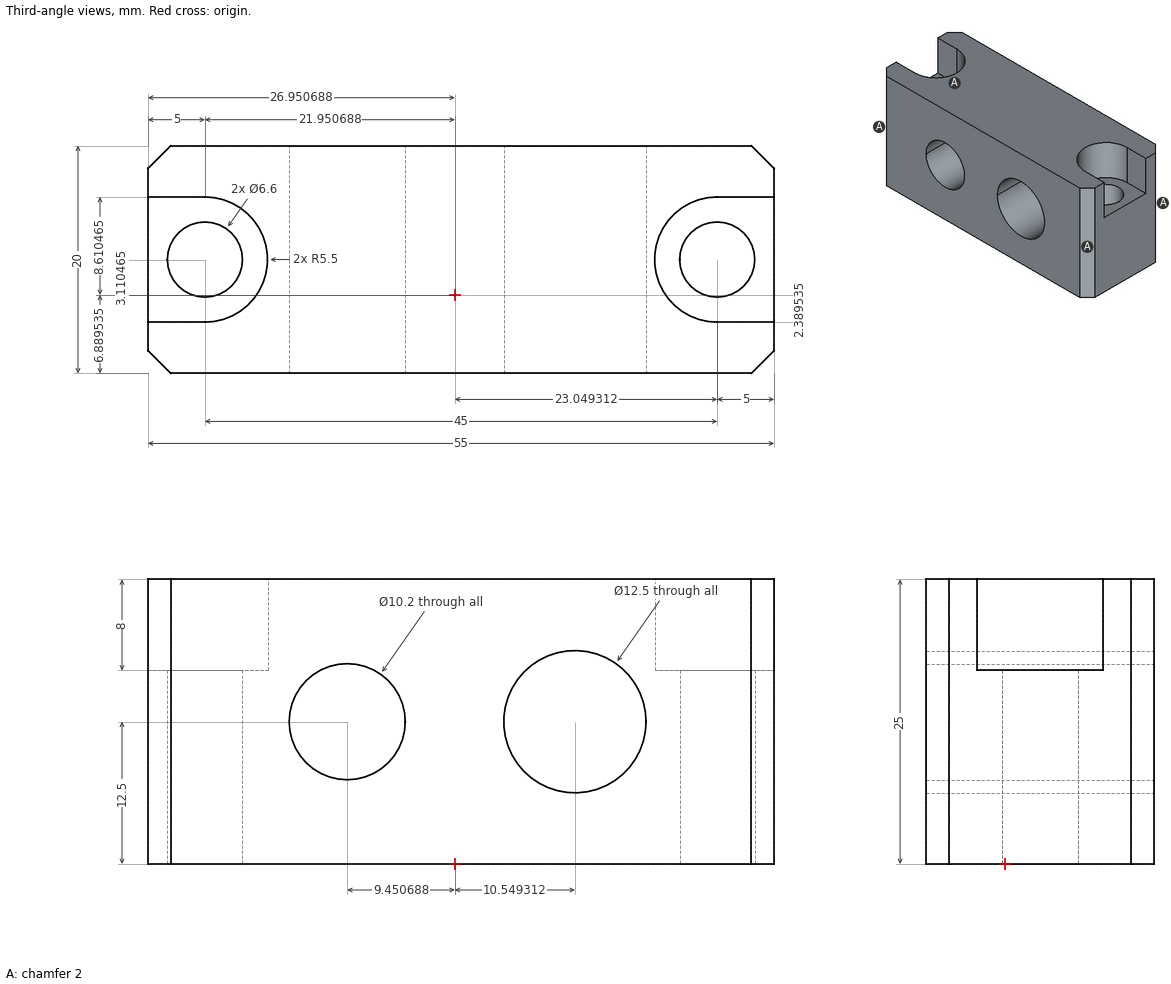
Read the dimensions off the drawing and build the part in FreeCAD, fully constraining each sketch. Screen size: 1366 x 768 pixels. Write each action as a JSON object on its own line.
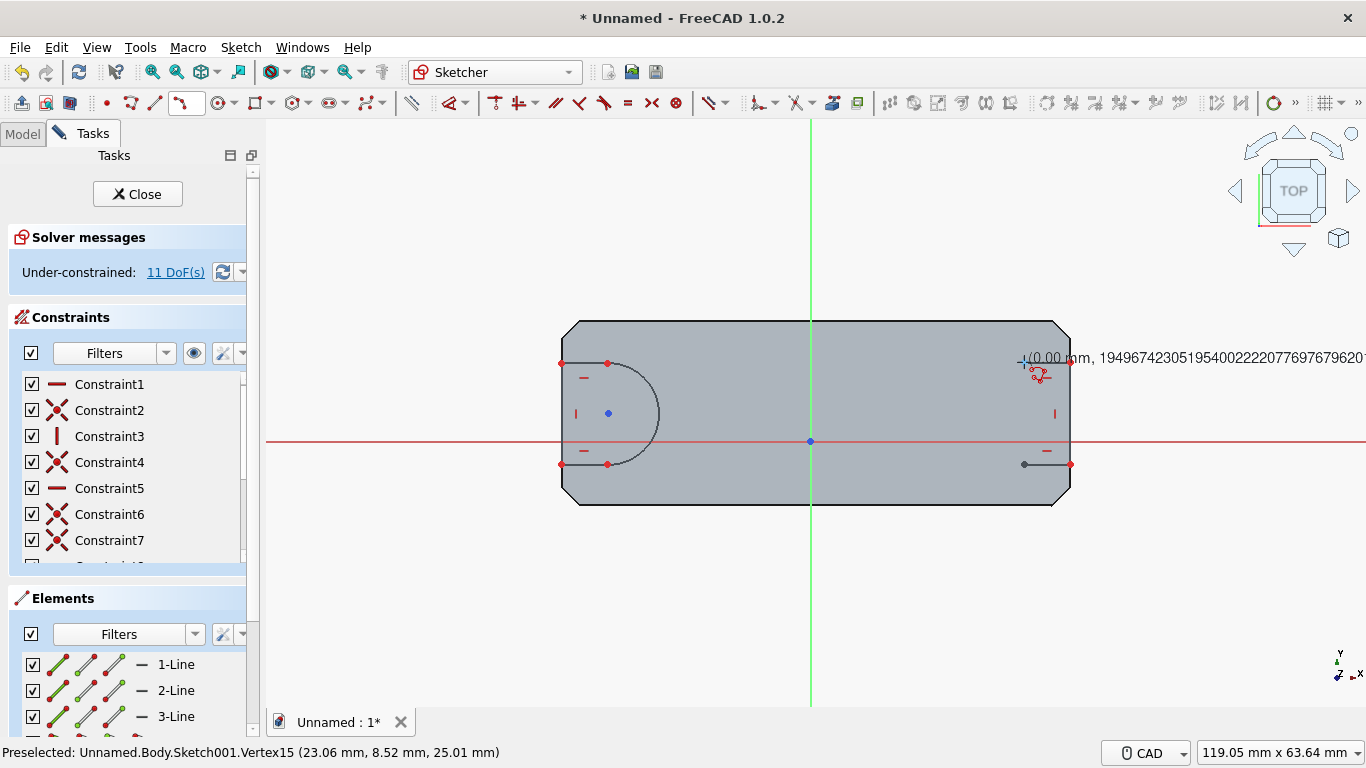
{"action": "key", "text": "g 3 a"}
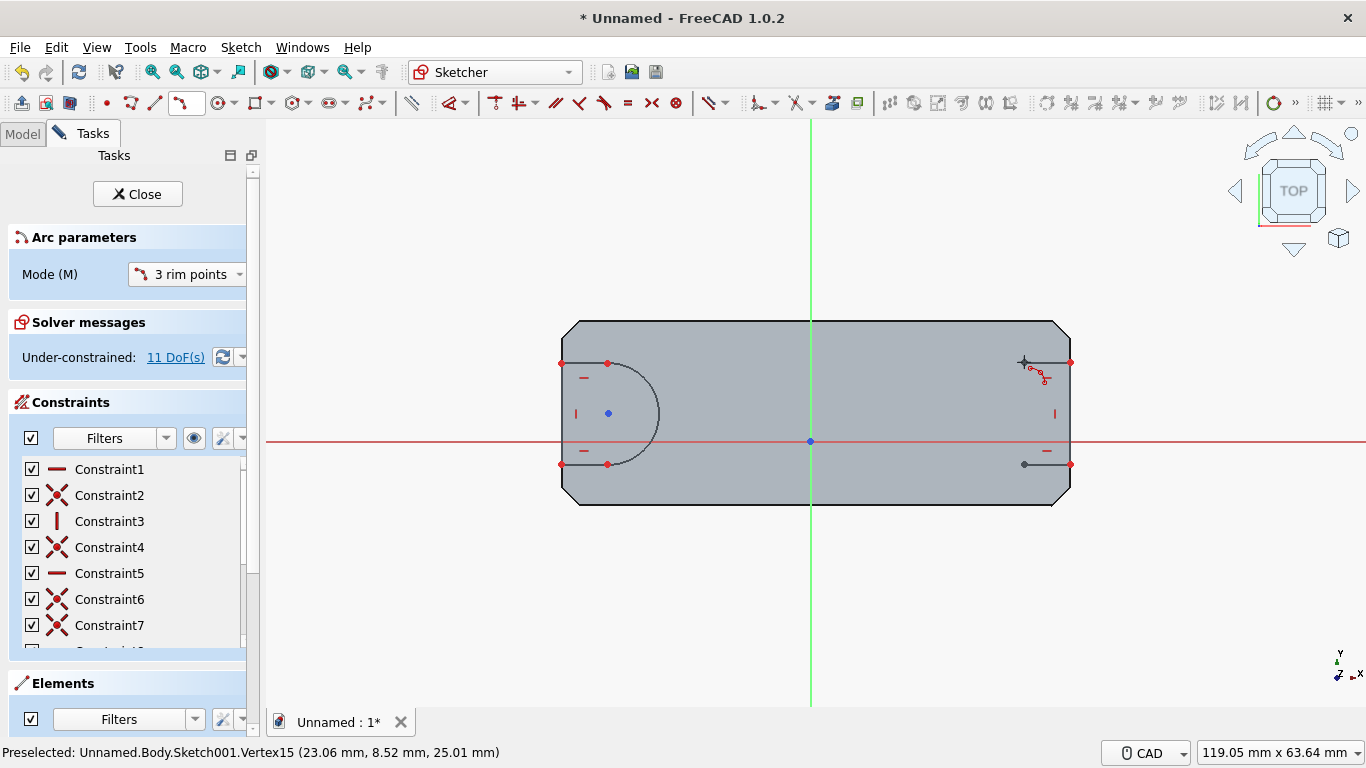
{"action": "left_click", "coordinate": [1024, 363]}
{"action": "left_click", "coordinate": [1024, 465]}
{"action": "left_click", "coordinate": [973, 413]}
{"action": "key", "text": "Escape"}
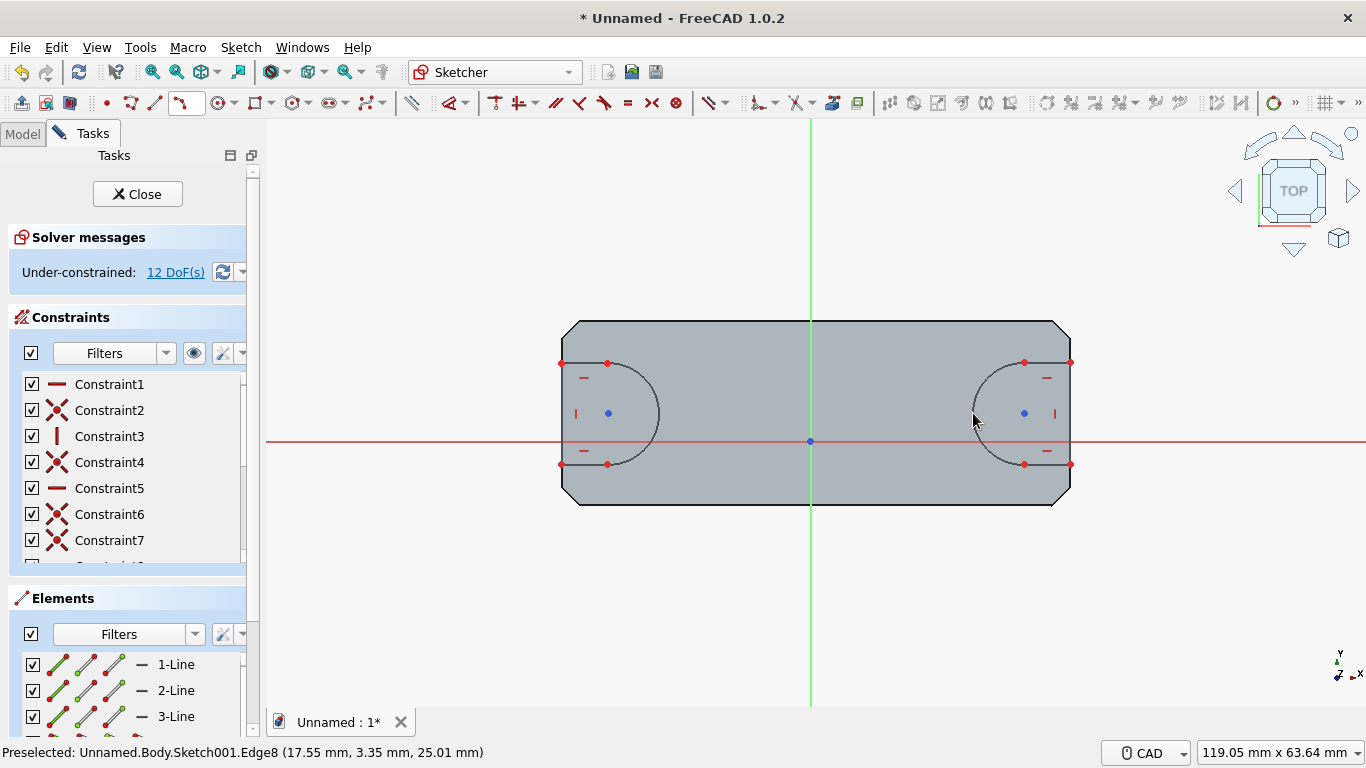
{"action": "left_click", "coordinate": [594, 363]}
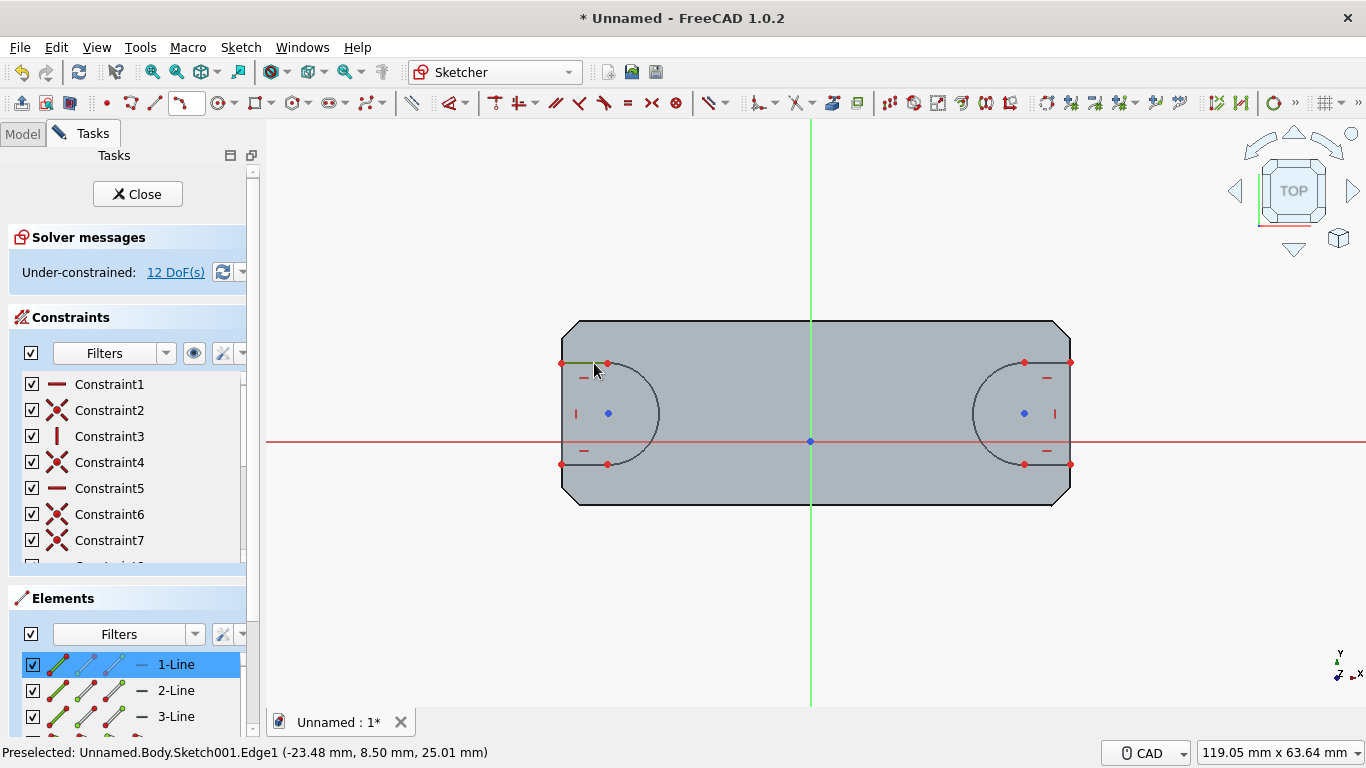
{"action": "left_click", "coordinate": [649, 444]}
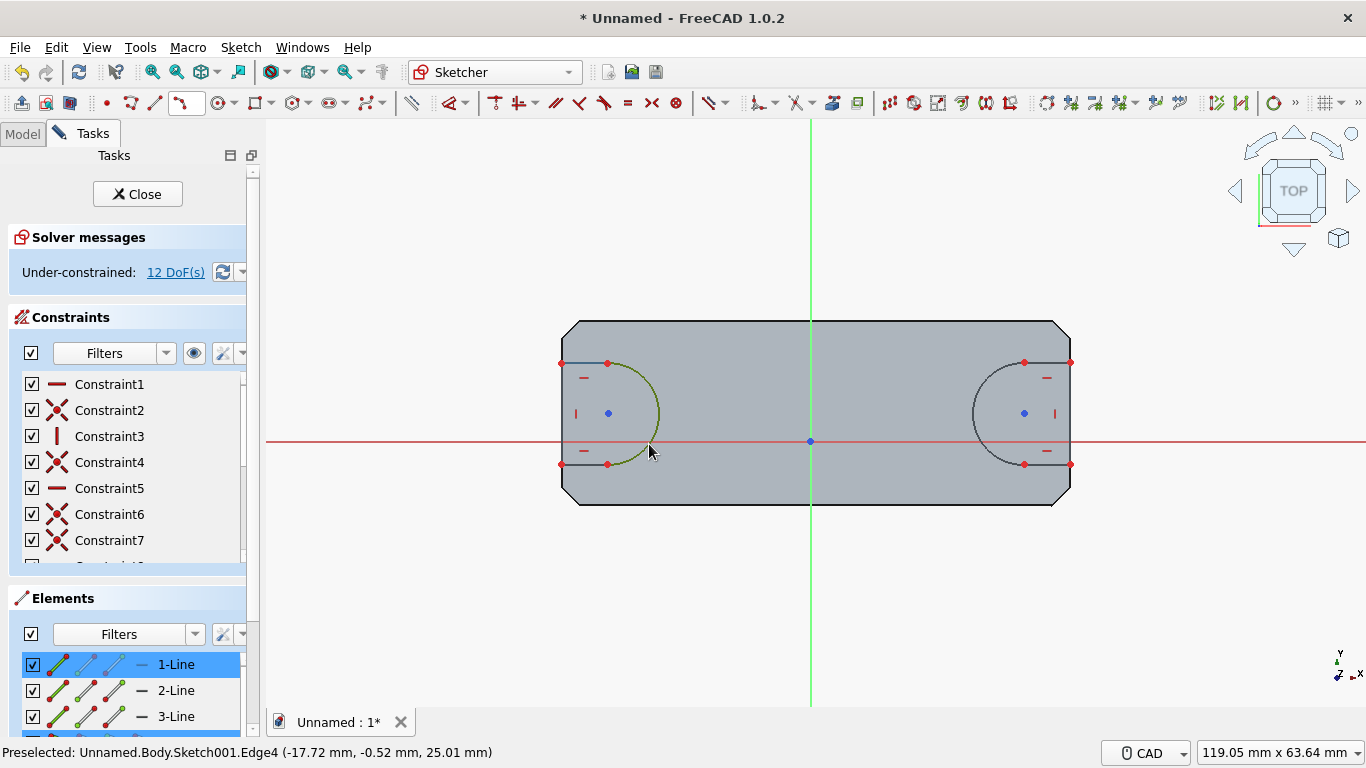
{"action": "key", "text": "t"}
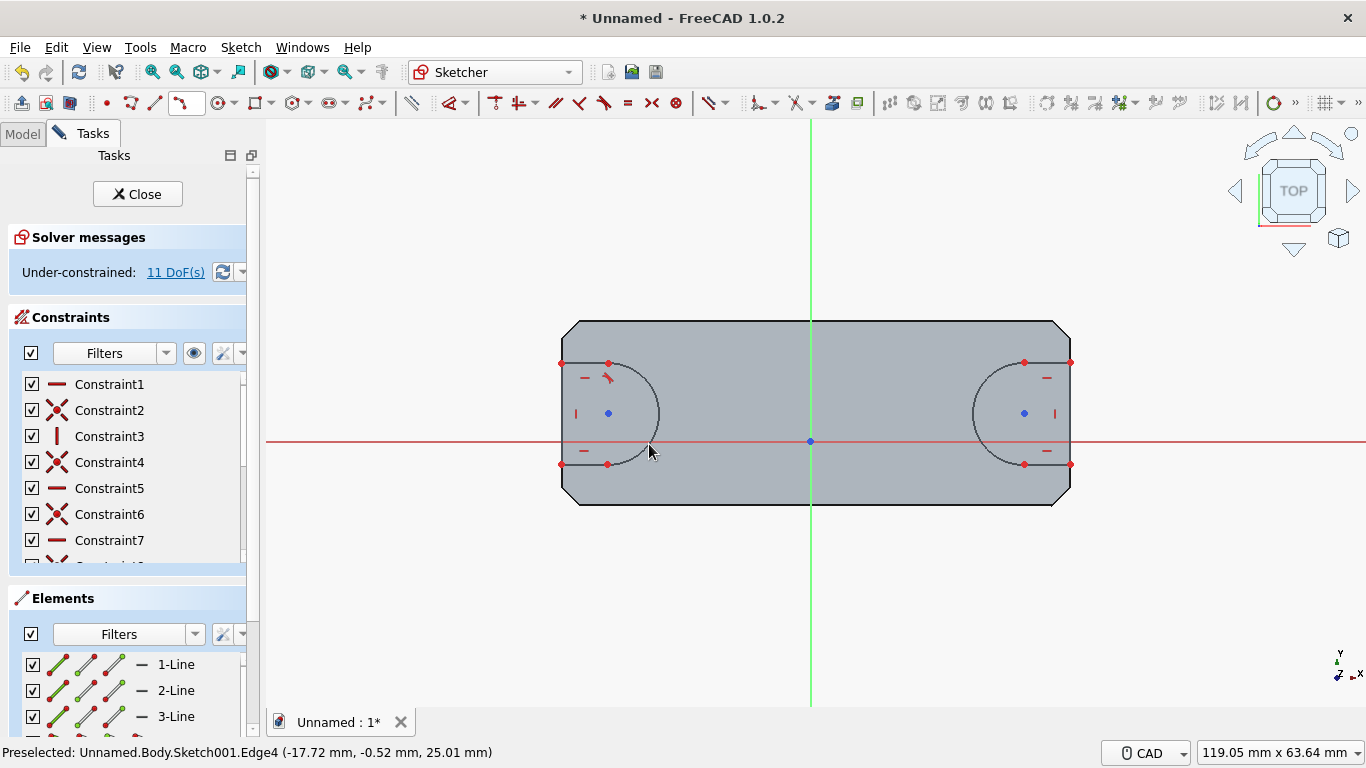
{"action": "left_click", "coordinate": [576, 465]}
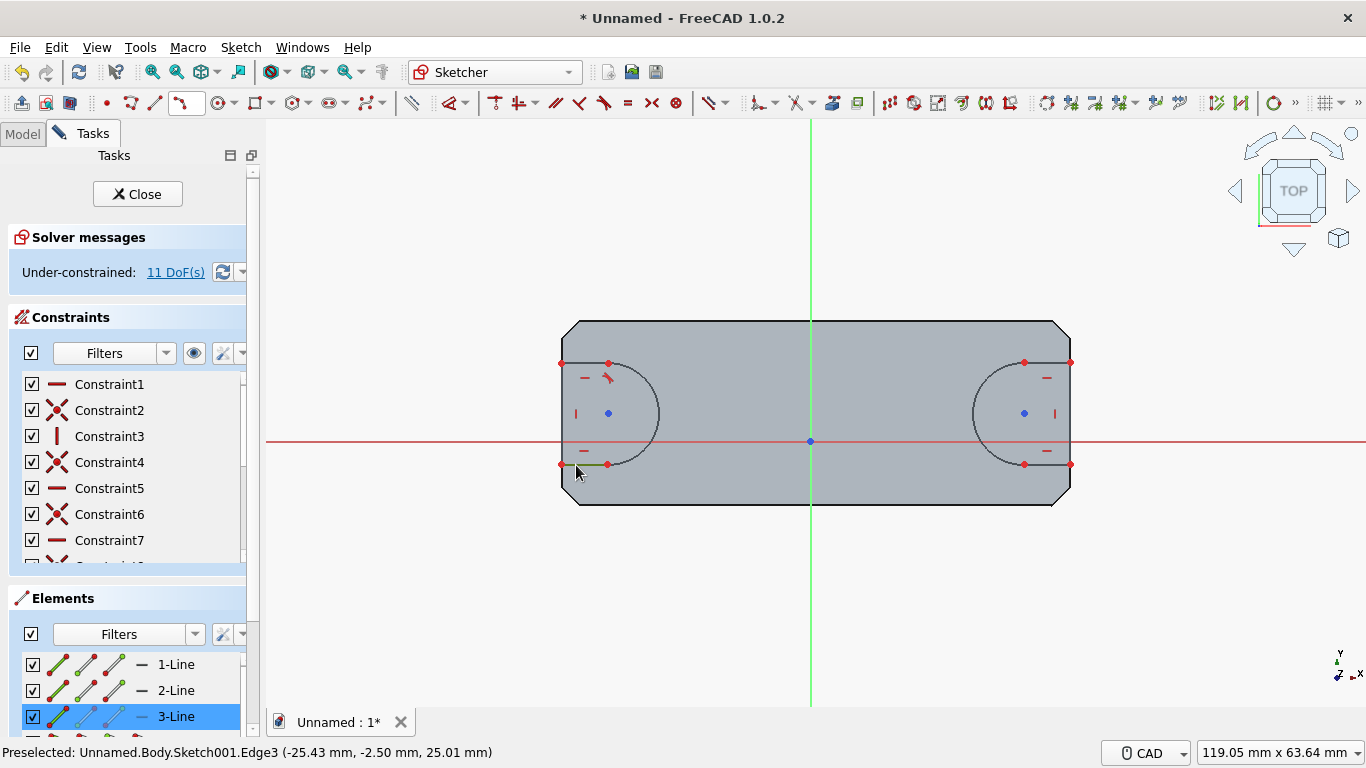
{"action": "left_click", "coordinate": [649, 444]}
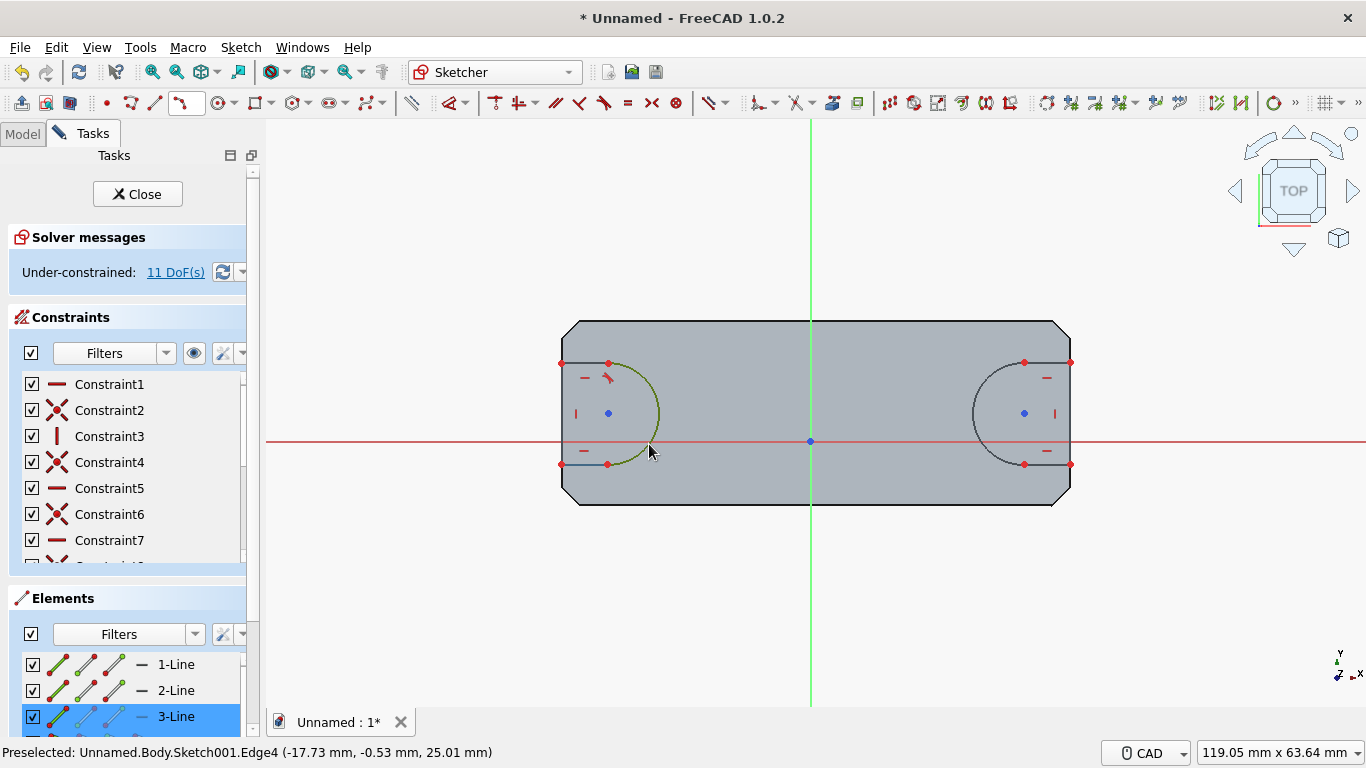
{"action": "key", "text": "t"}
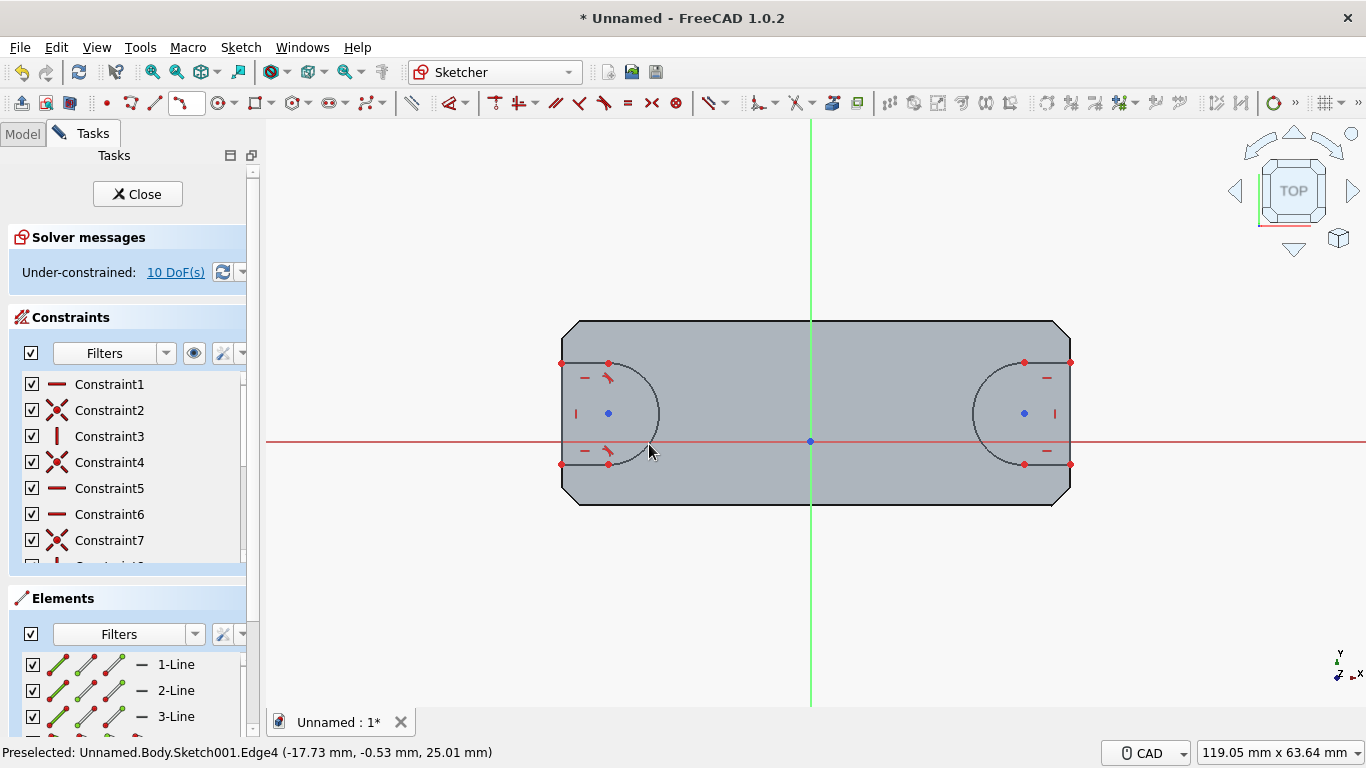
{"action": "left_click", "coordinate": [1038, 465]}